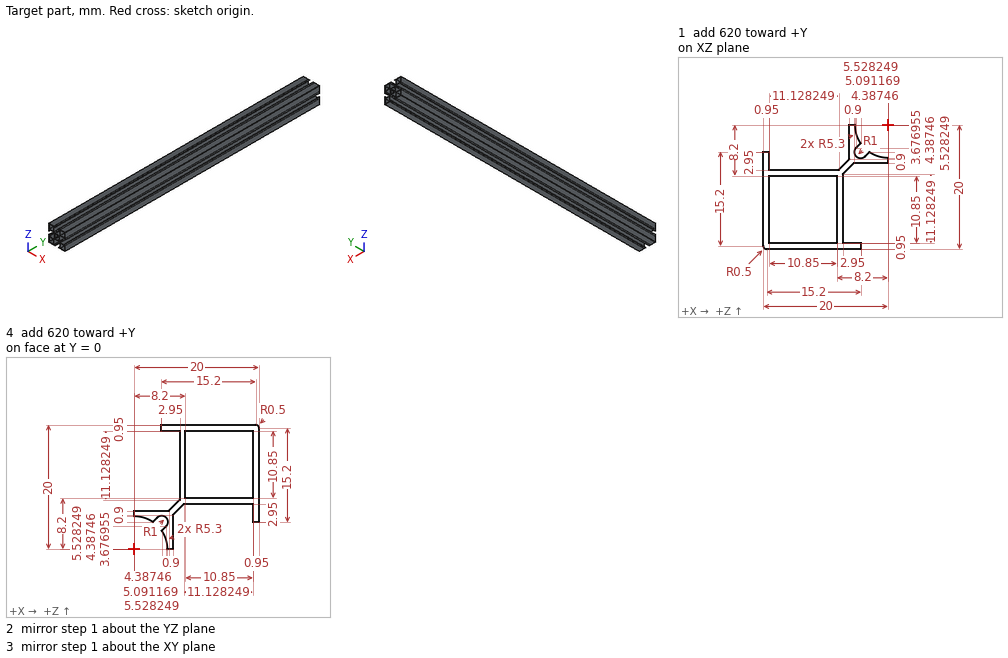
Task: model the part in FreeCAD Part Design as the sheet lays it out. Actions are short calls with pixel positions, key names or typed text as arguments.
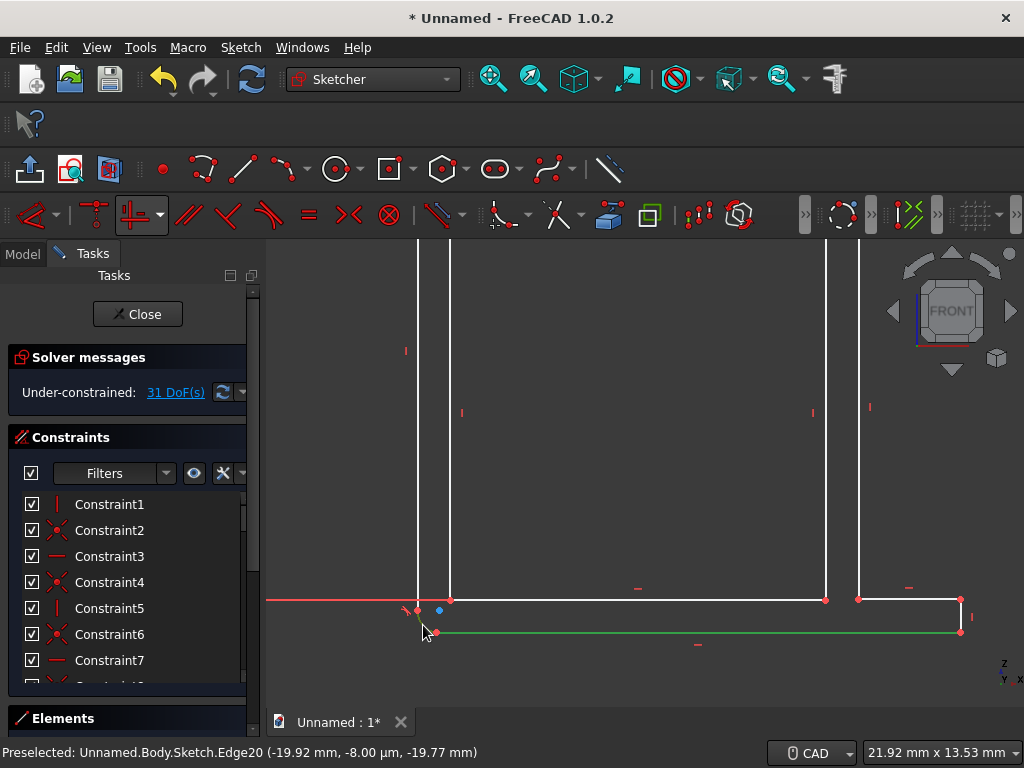
click(270, 216)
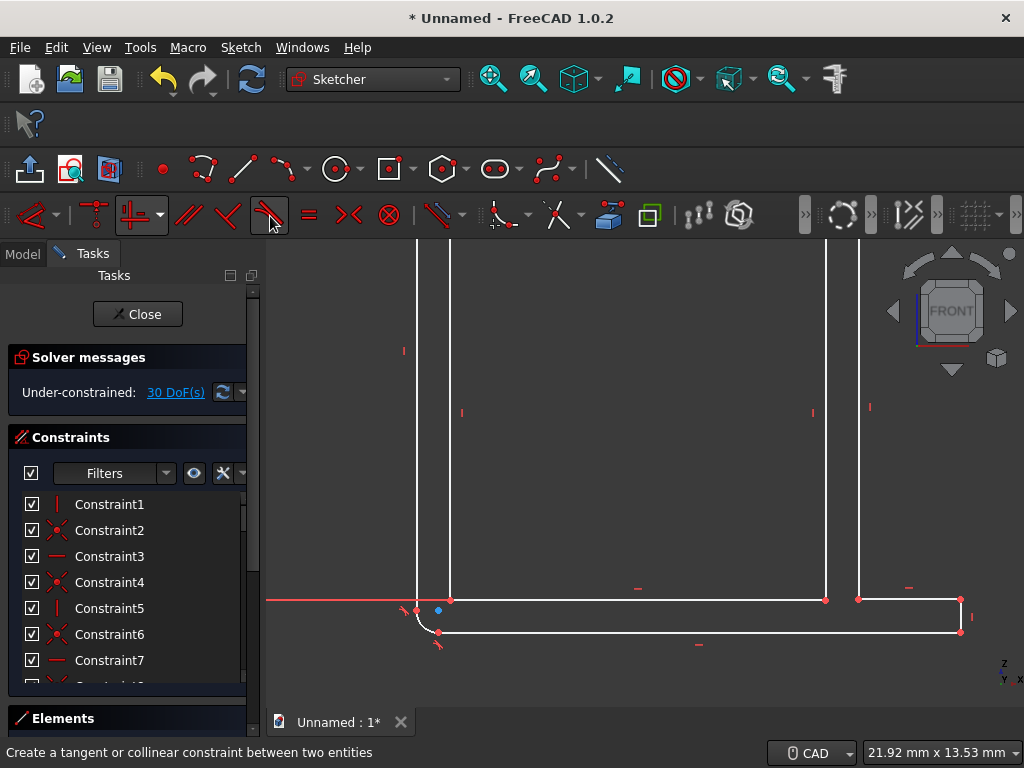
scroll(424, 627, down, 4)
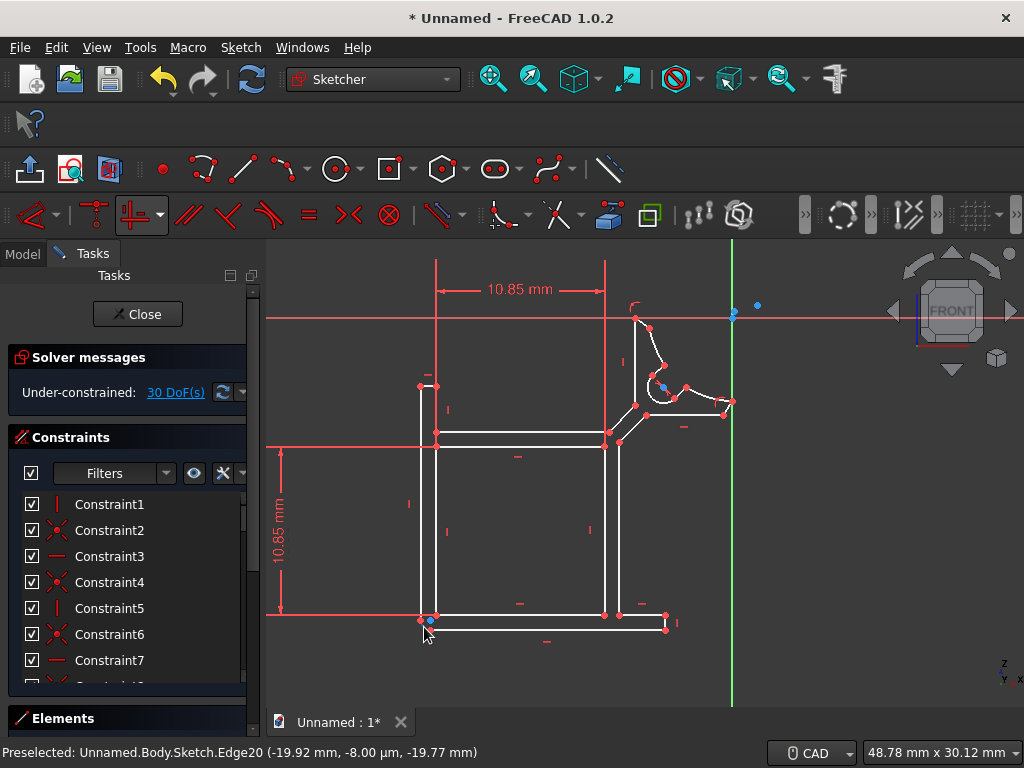
scroll(645, 325, up, 5)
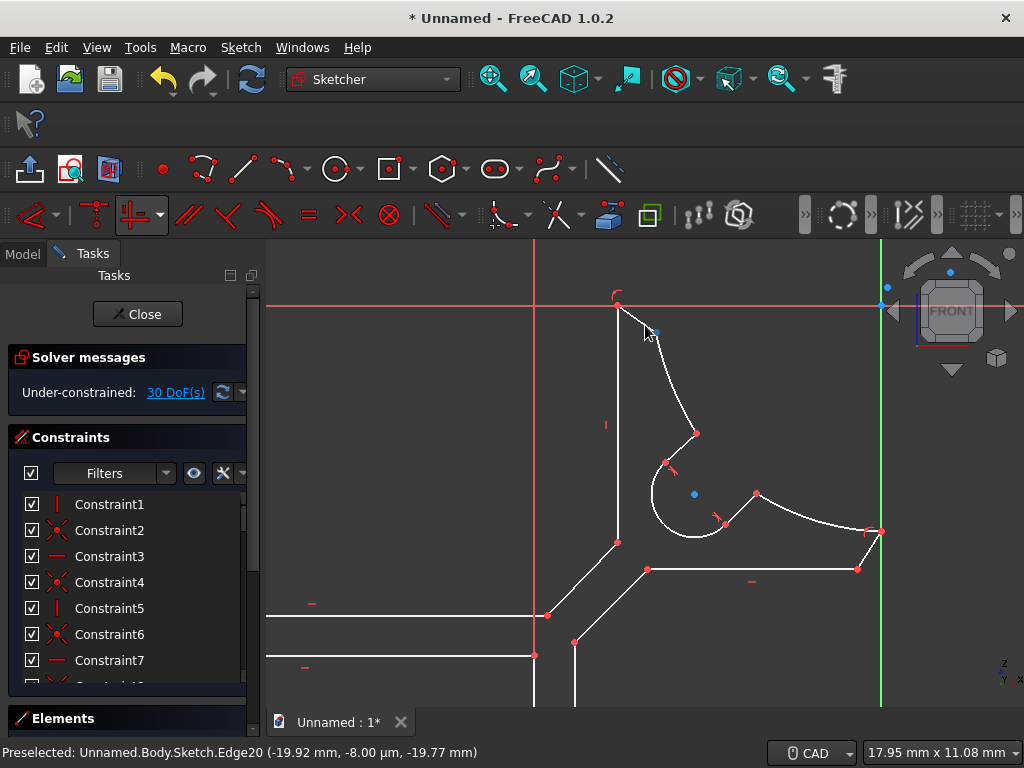
click(645, 325)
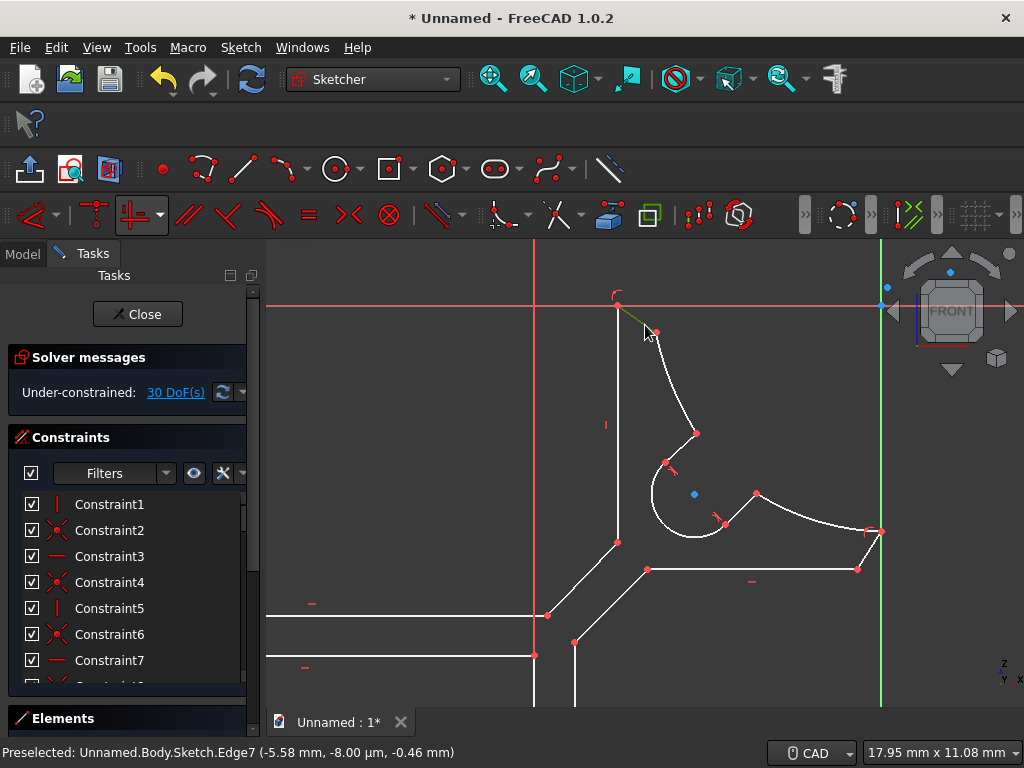
click(162, 216)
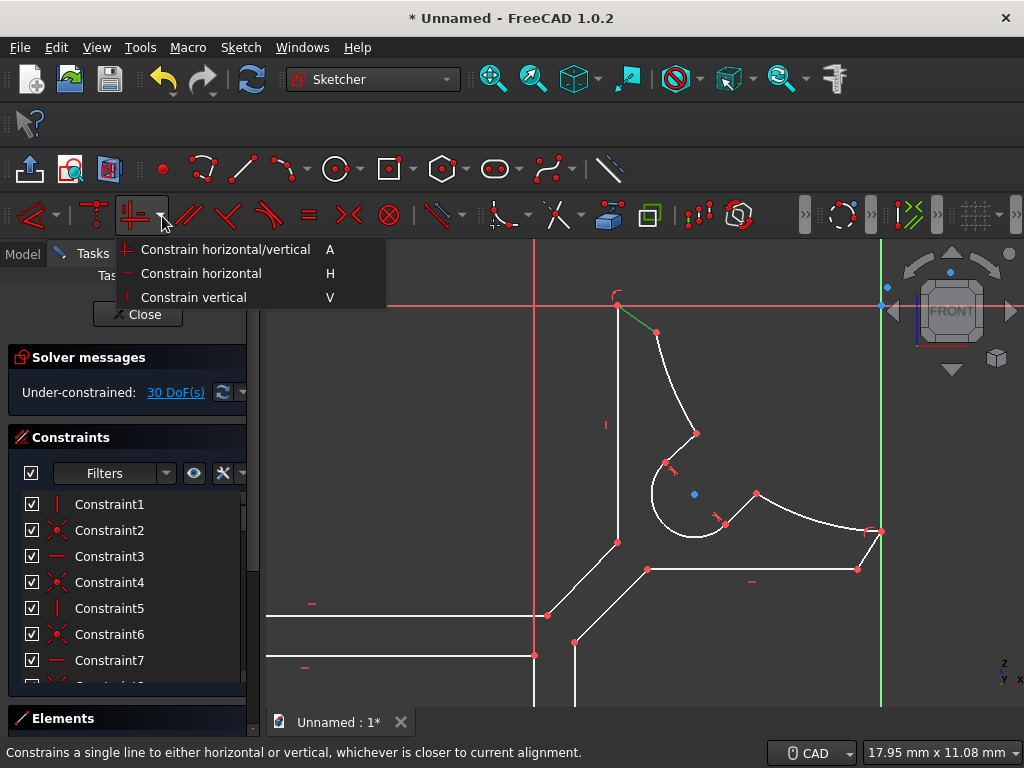
click(251, 273)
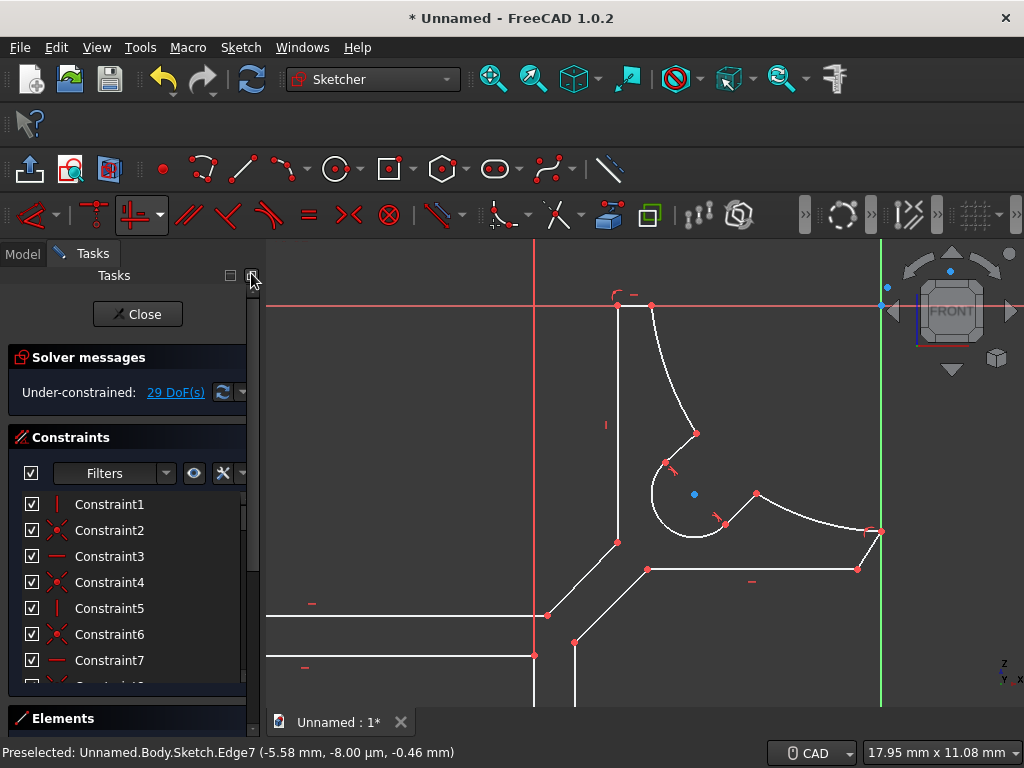
scroll(645, 324, down, 5)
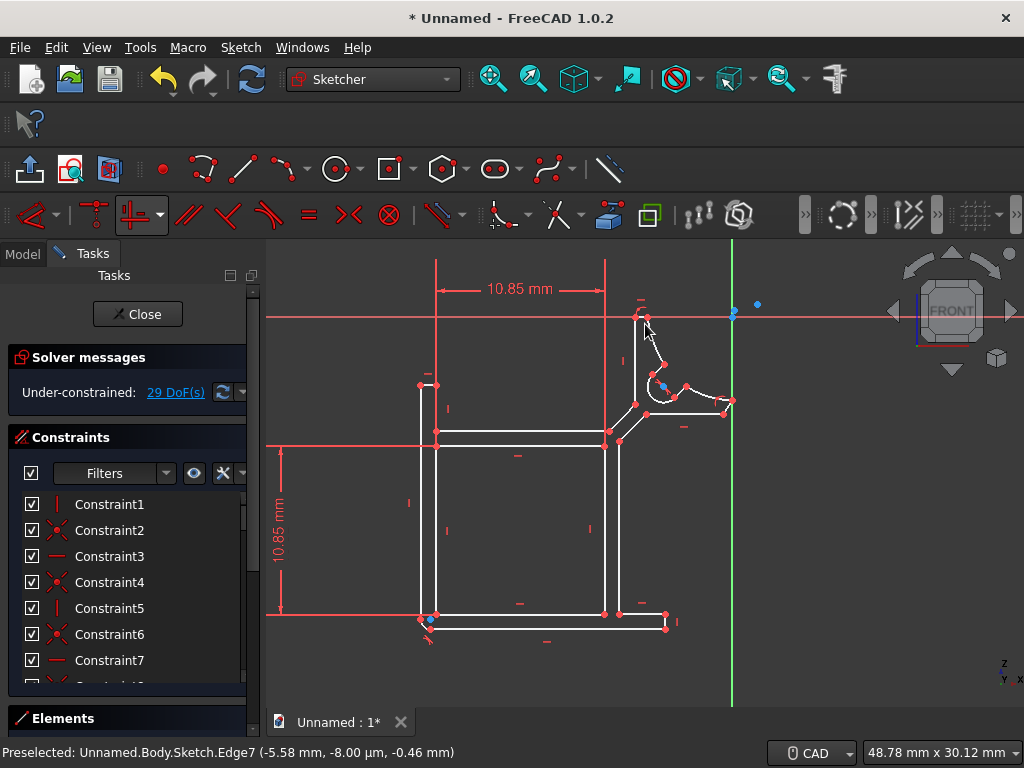
scroll(726, 410, up, 6)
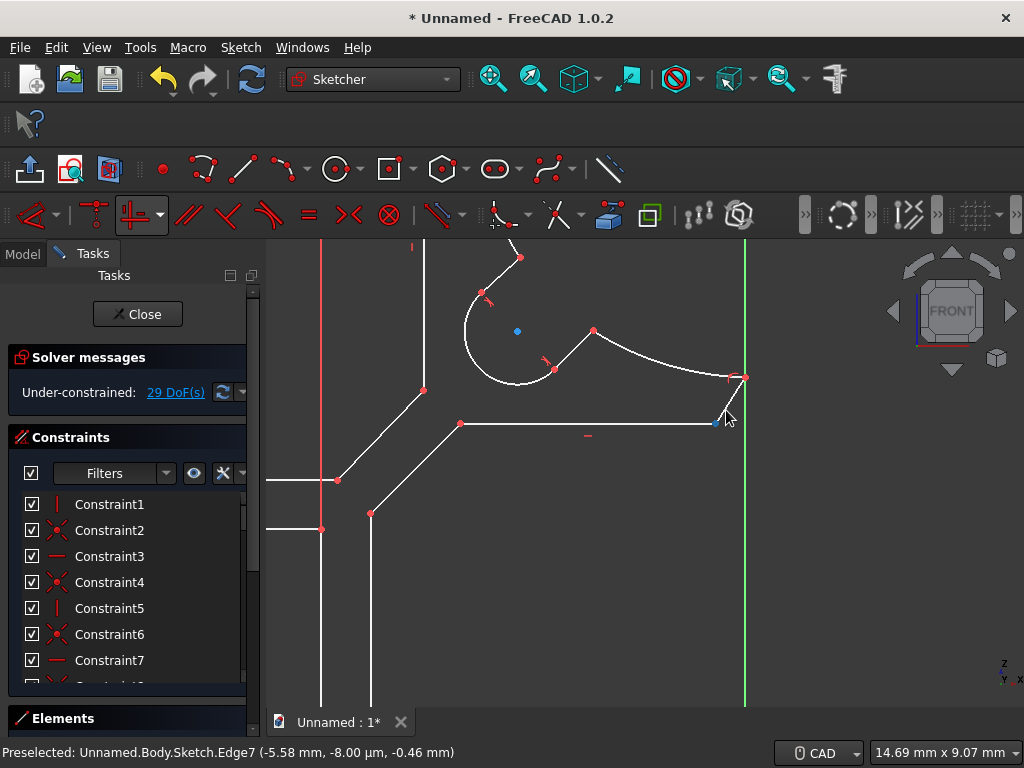
click(725, 410)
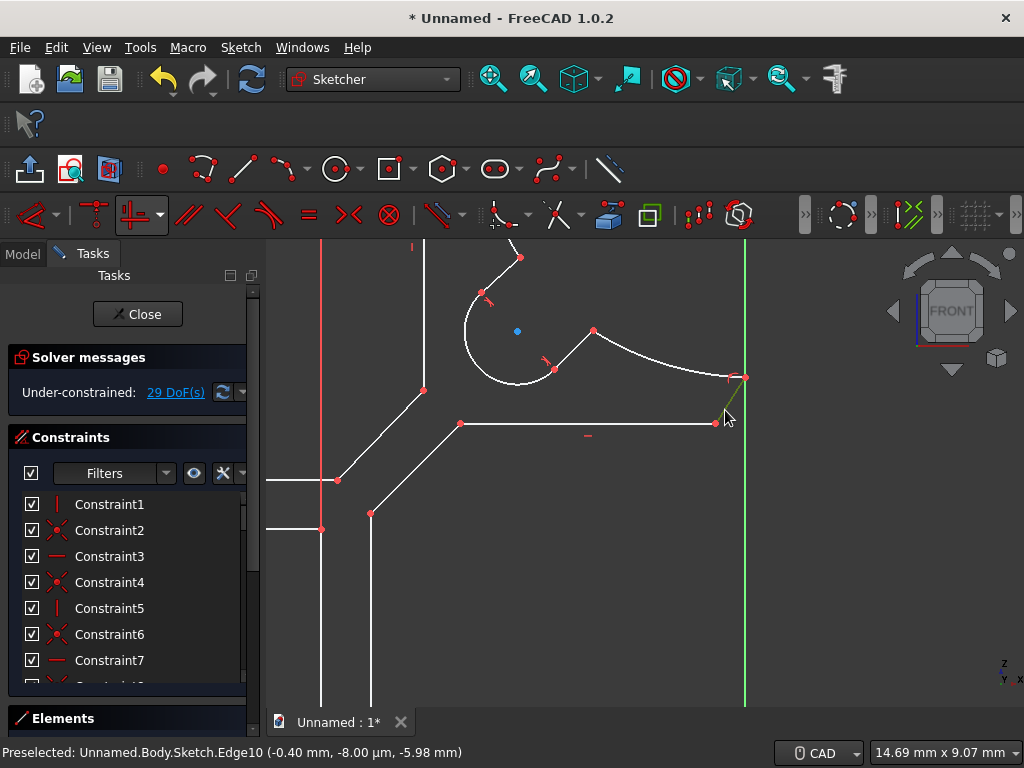
click(162, 216)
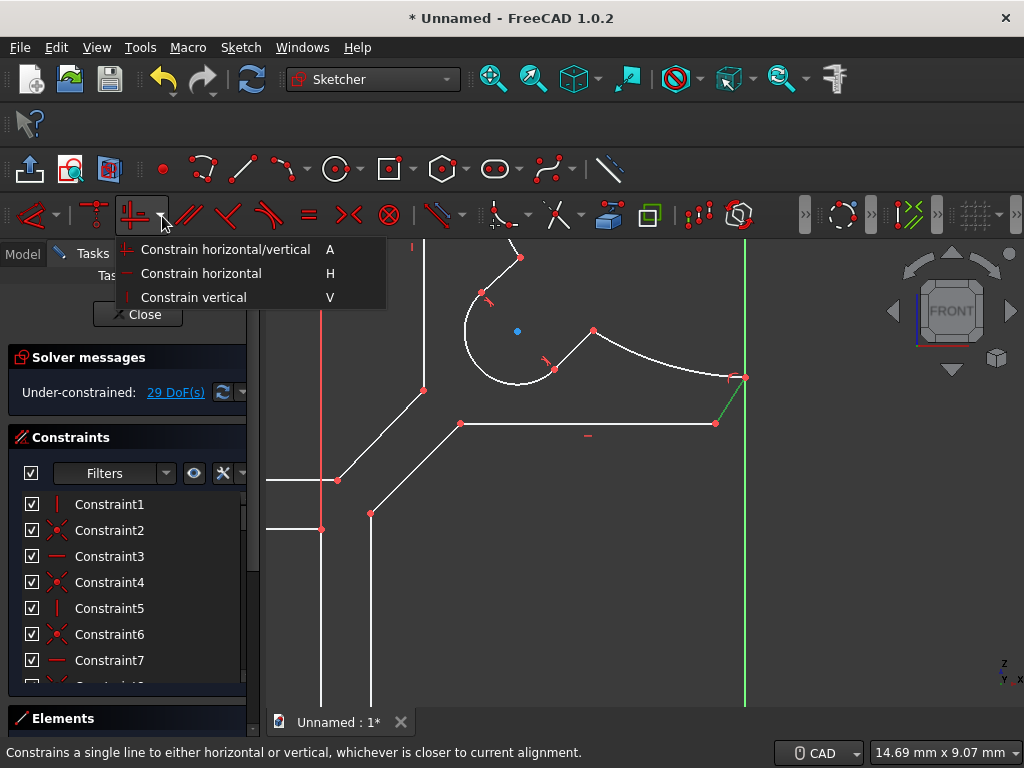
click(251, 297)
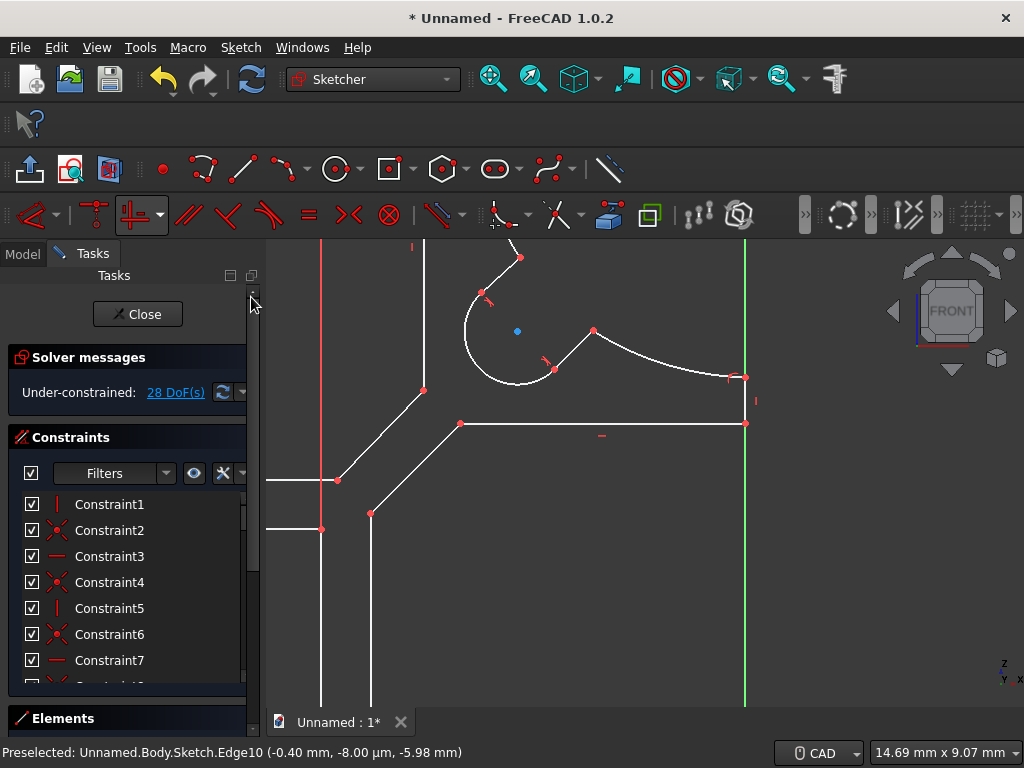
scroll(726, 411, down, 6)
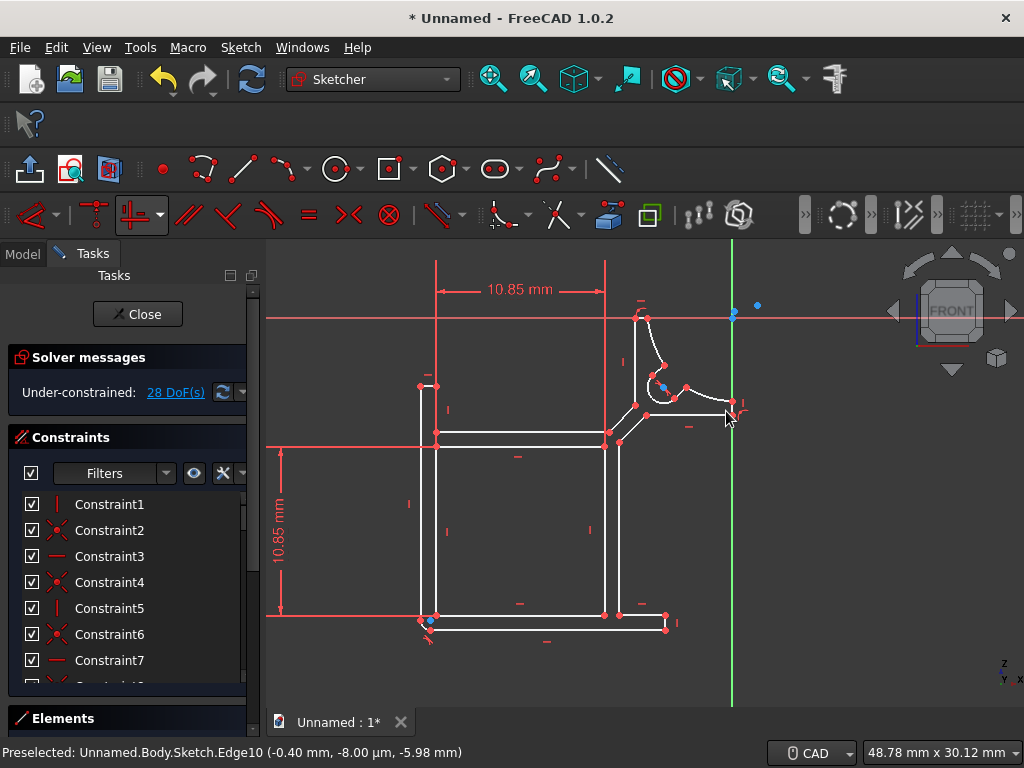
click(650, 333)